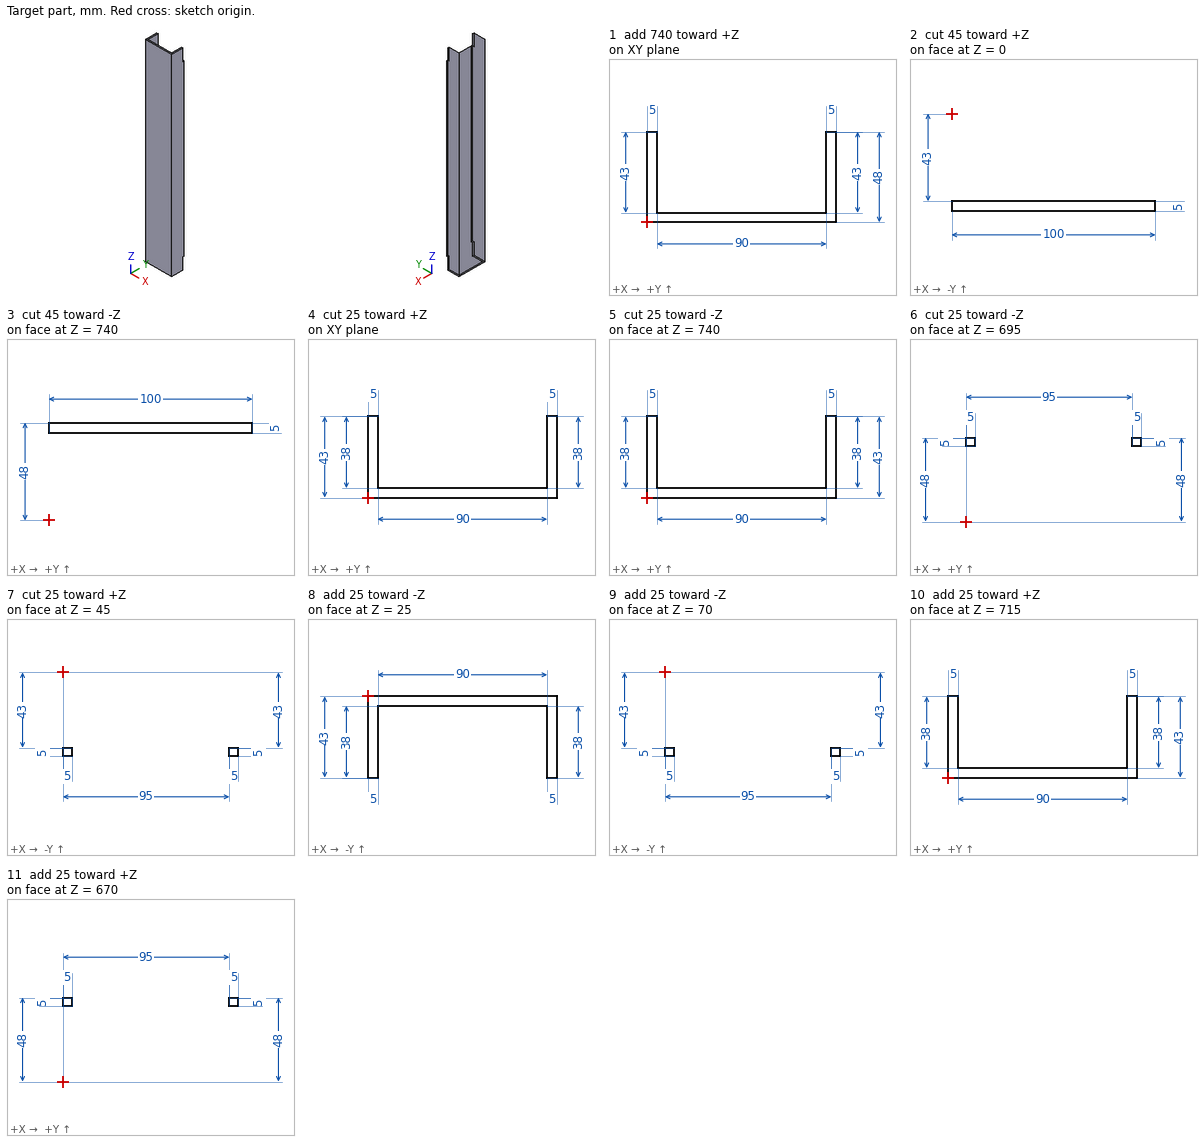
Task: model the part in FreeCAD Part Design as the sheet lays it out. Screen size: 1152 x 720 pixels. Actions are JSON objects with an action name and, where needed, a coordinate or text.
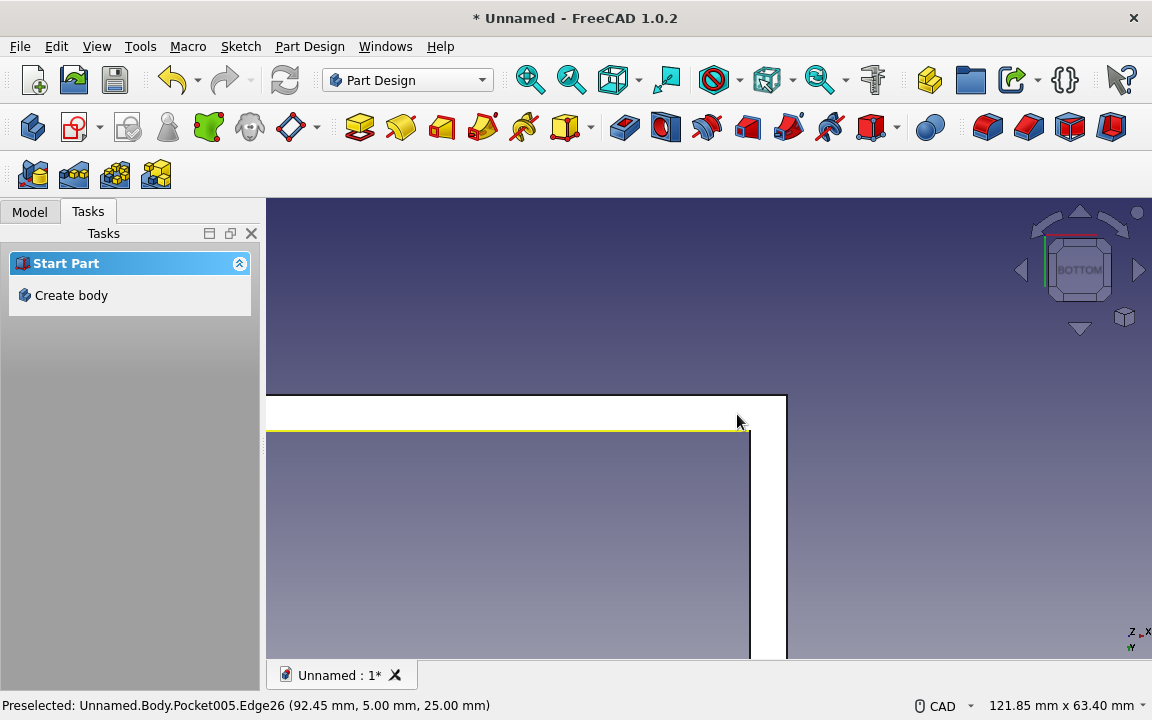
{"action": "left_click", "coordinate": [735, 416]}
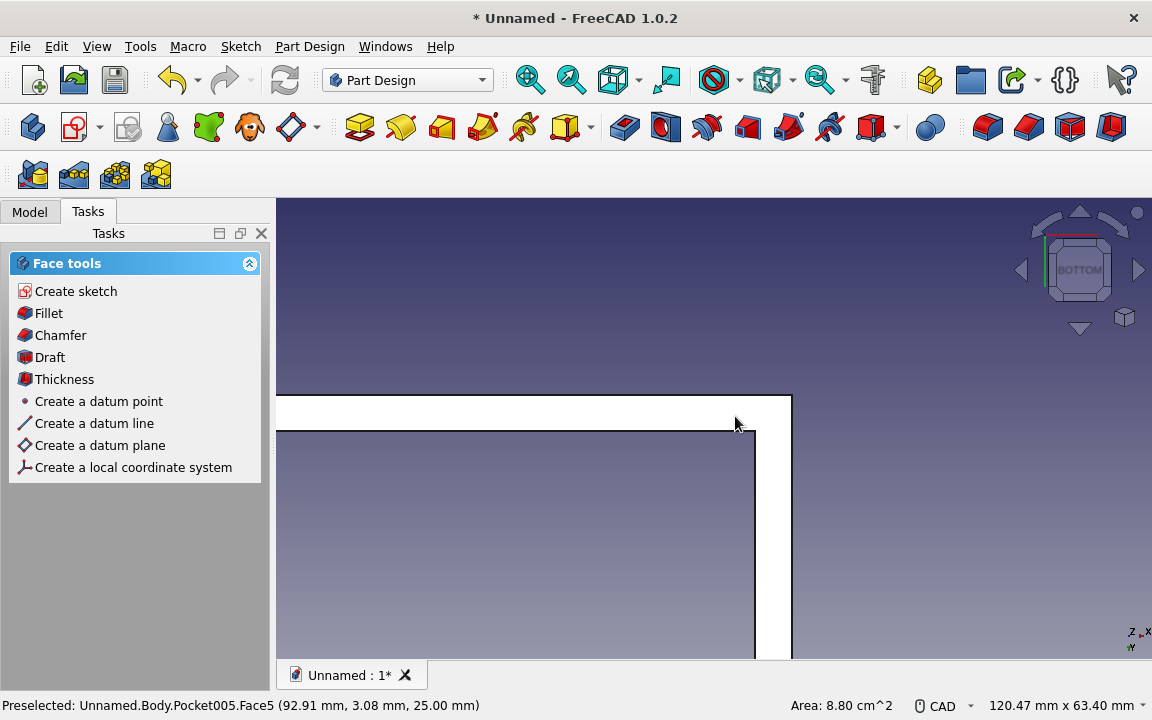
{"action": "left_click", "coordinate": [74, 128]}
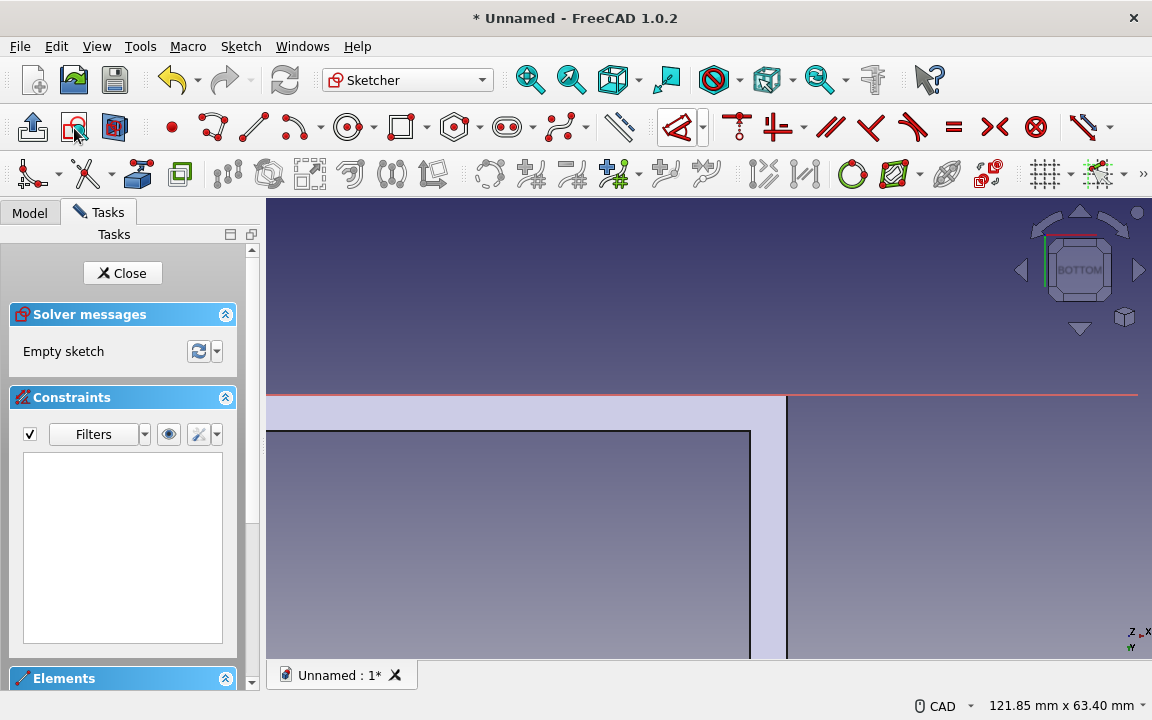
{"action": "scroll", "coordinate": [987, 226], "scroll_direction": "down", "scroll_amount": 2}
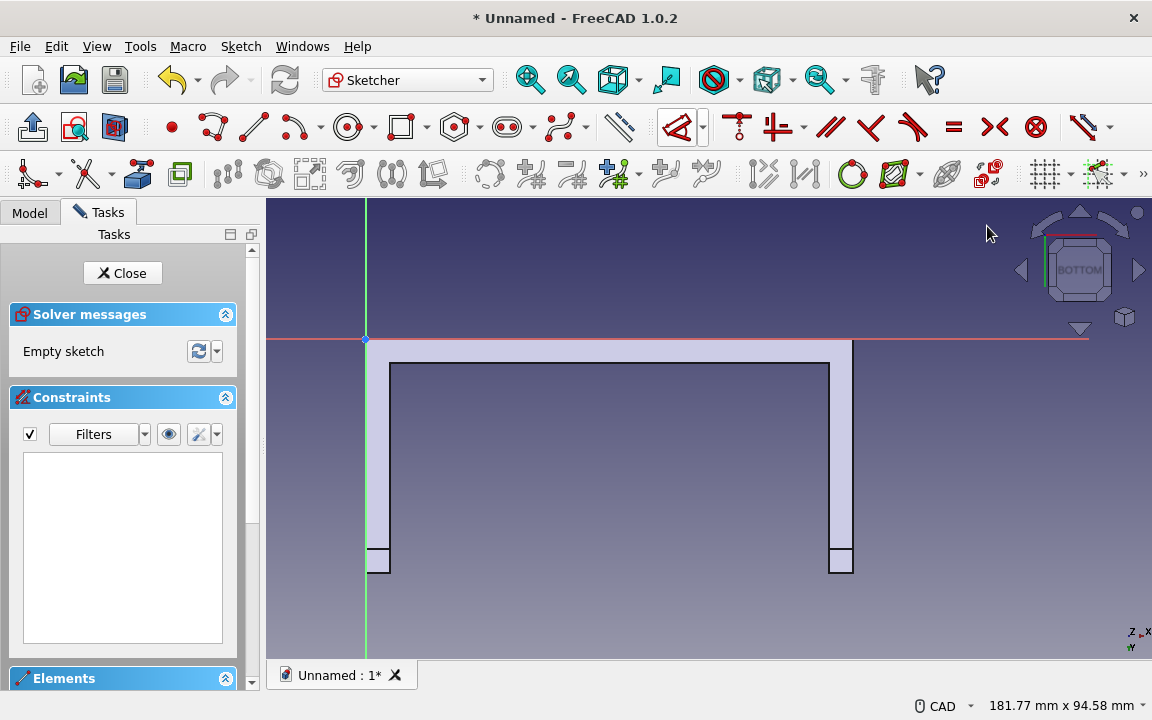
{"action": "left_click", "coordinate": [213, 128]}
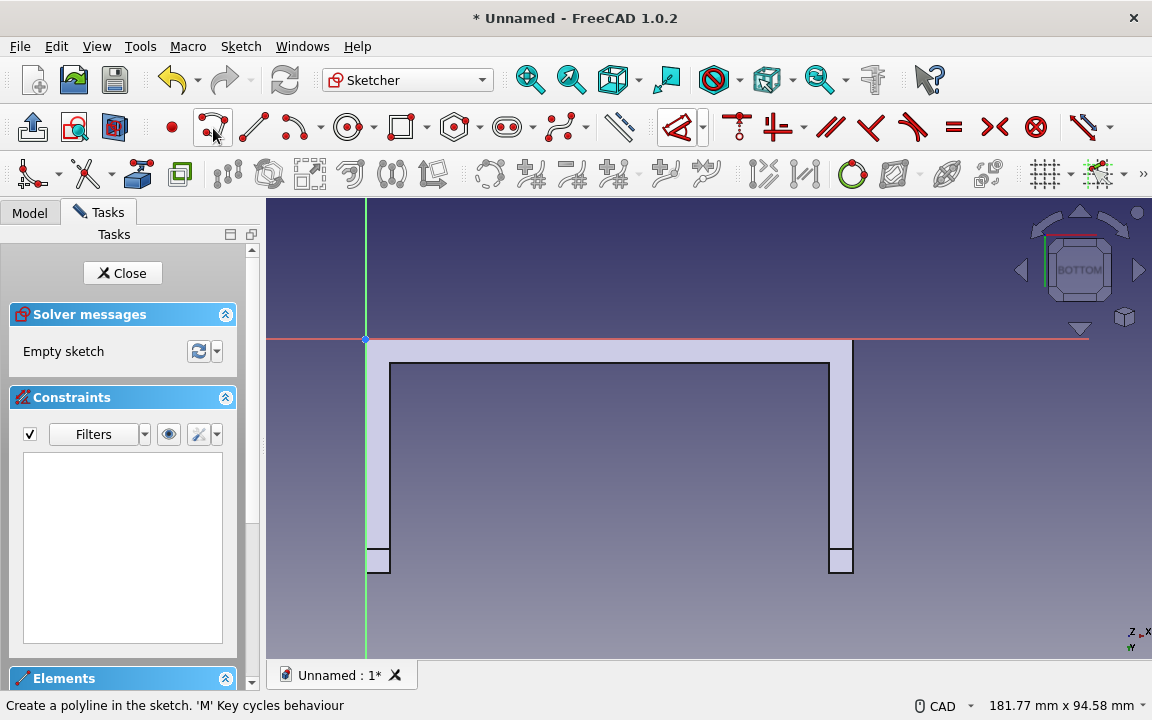
{"action": "left_click", "coordinate": [366, 339]}
{"action": "left_click", "coordinate": [375, 549]}
{"action": "left_click", "coordinate": [390, 549]}
{"action": "left_click", "coordinate": [390, 363]}
{"action": "left_click", "coordinate": [829, 363]}
{"action": "left_click", "coordinate": [829, 549]}
{"action": "left_click", "coordinate": [853, 549]}
{"action": "left_click", "coordinate": [853, 348]}
{"action": "left_click", "coordinate": [366, 339]}
{"action": "key", "text": "Escape"}
{"action": "key", "text": "Escape"}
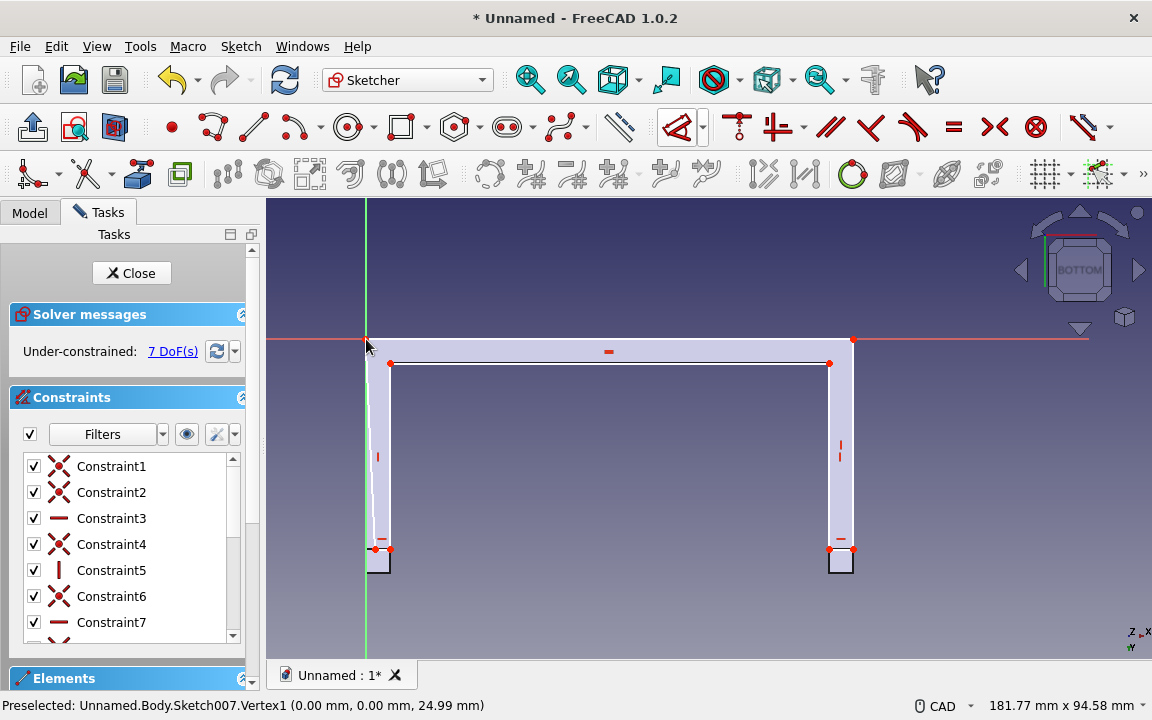
{"action": "left_click", "coordinate": [368, 402]}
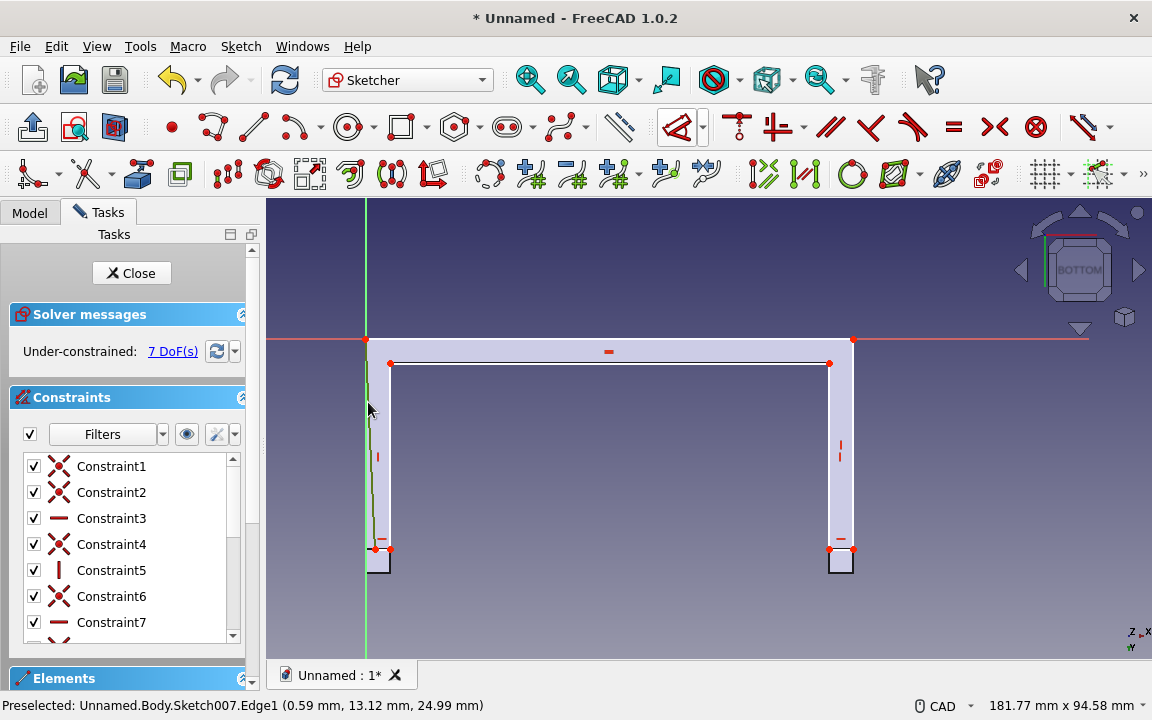
{"action": "left_click", "coordinate": [804, 128]}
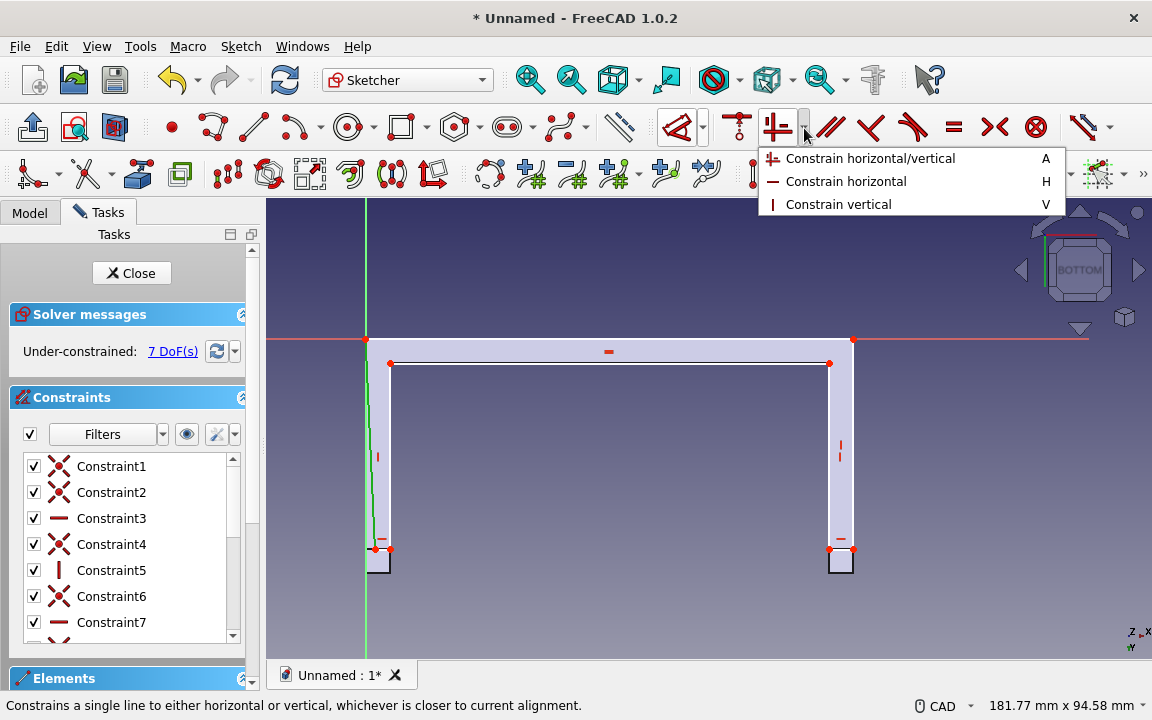
{"action": "left_click", "coordinate": [912, 204]}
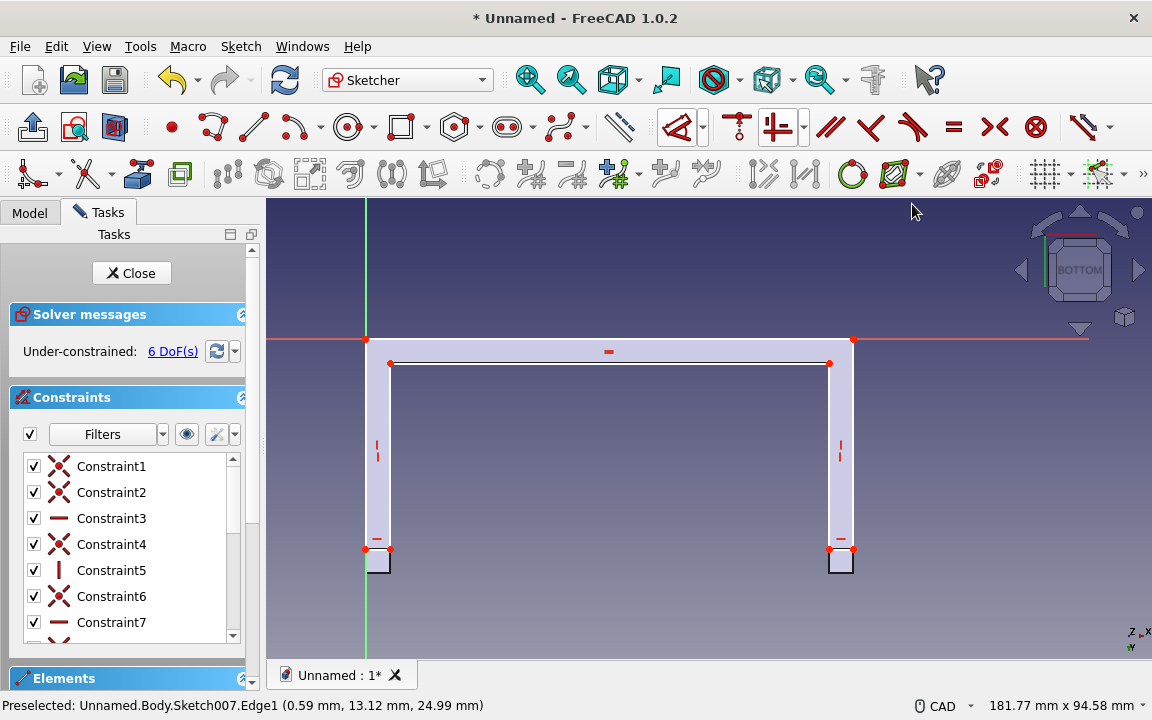
{"action": "scroll", "coordinate": [375, 550], "scroll_direction": "up", "scroll_amount": 3}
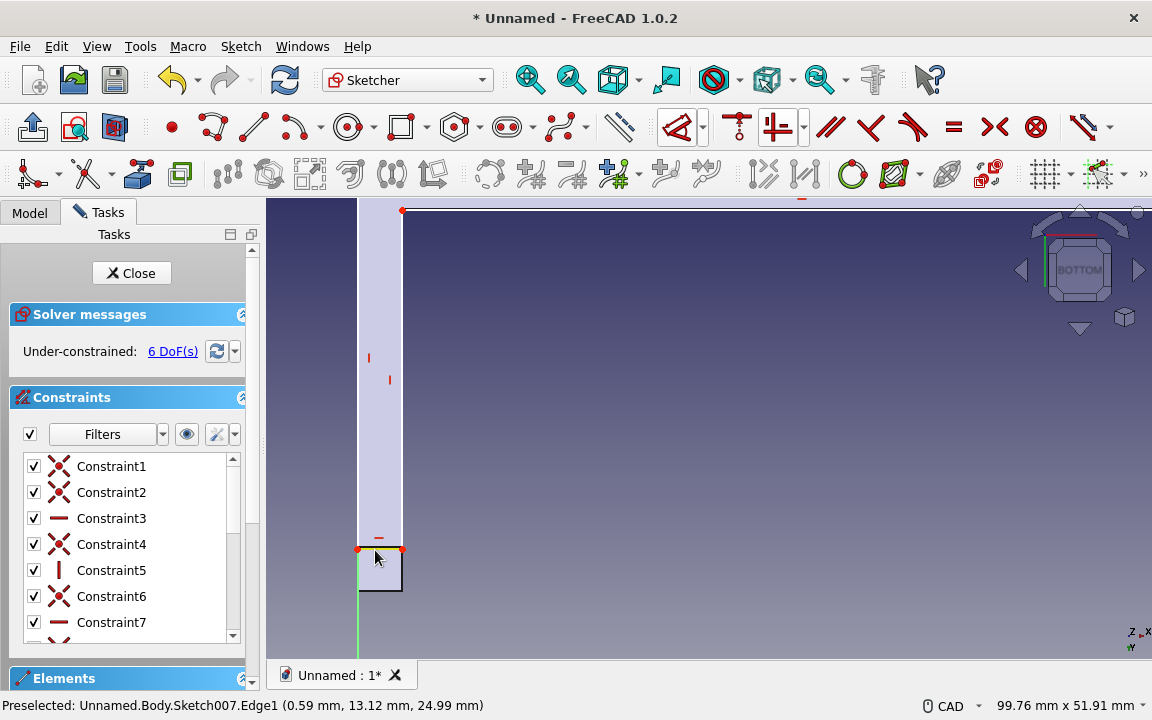
{"action": "left_click", "coordinate": [375, 549]}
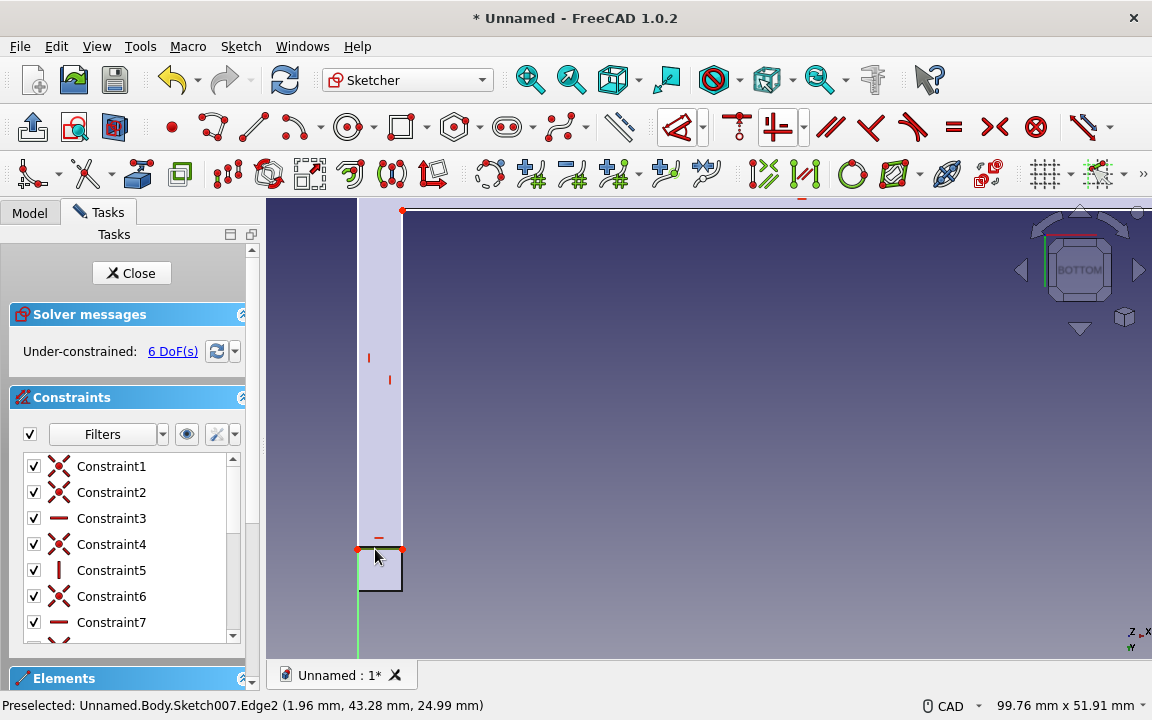
{"action": "key", "text": "l"}